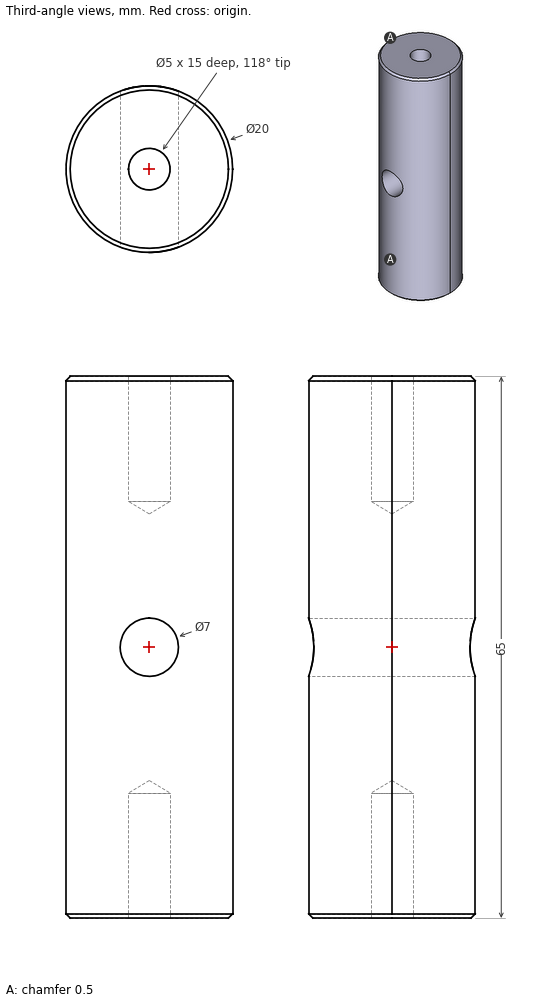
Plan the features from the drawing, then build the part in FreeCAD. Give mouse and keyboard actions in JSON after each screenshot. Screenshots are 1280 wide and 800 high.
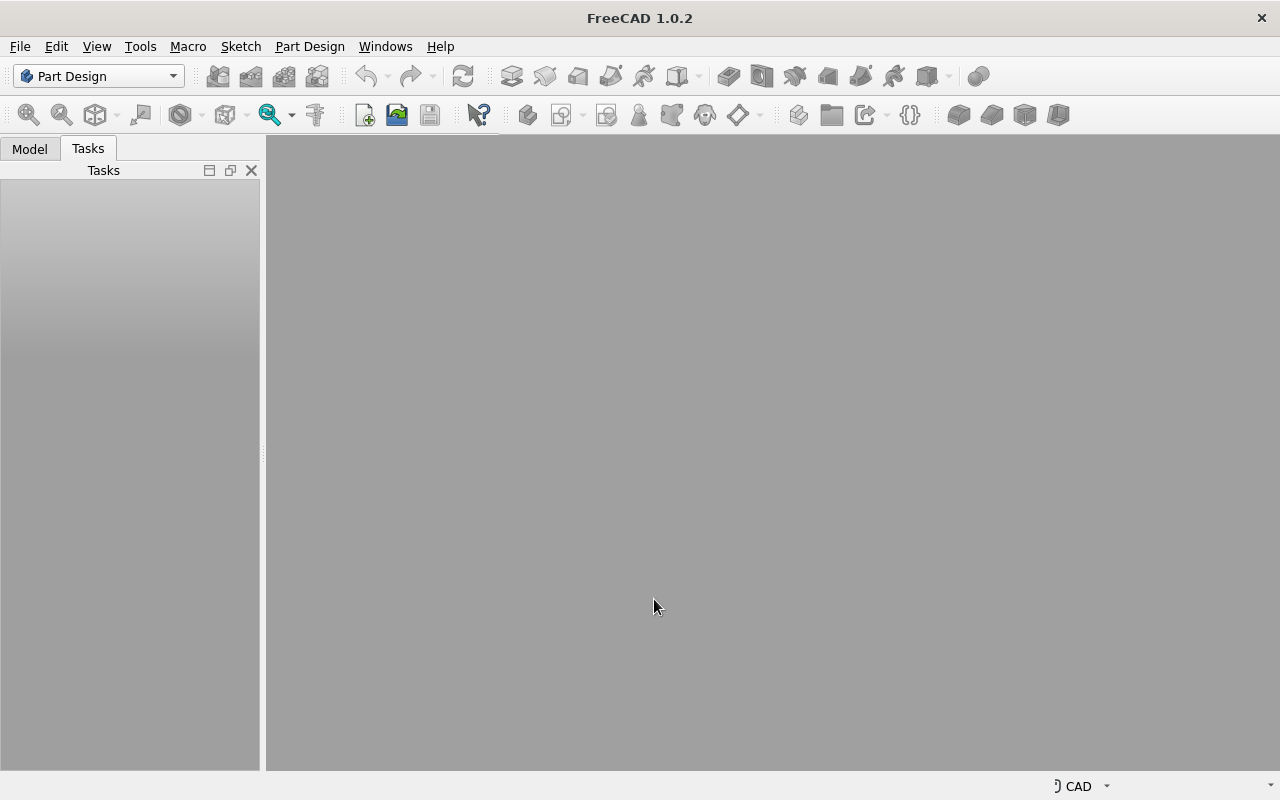
{"action": "left_click", "coordinate": [364, 116]}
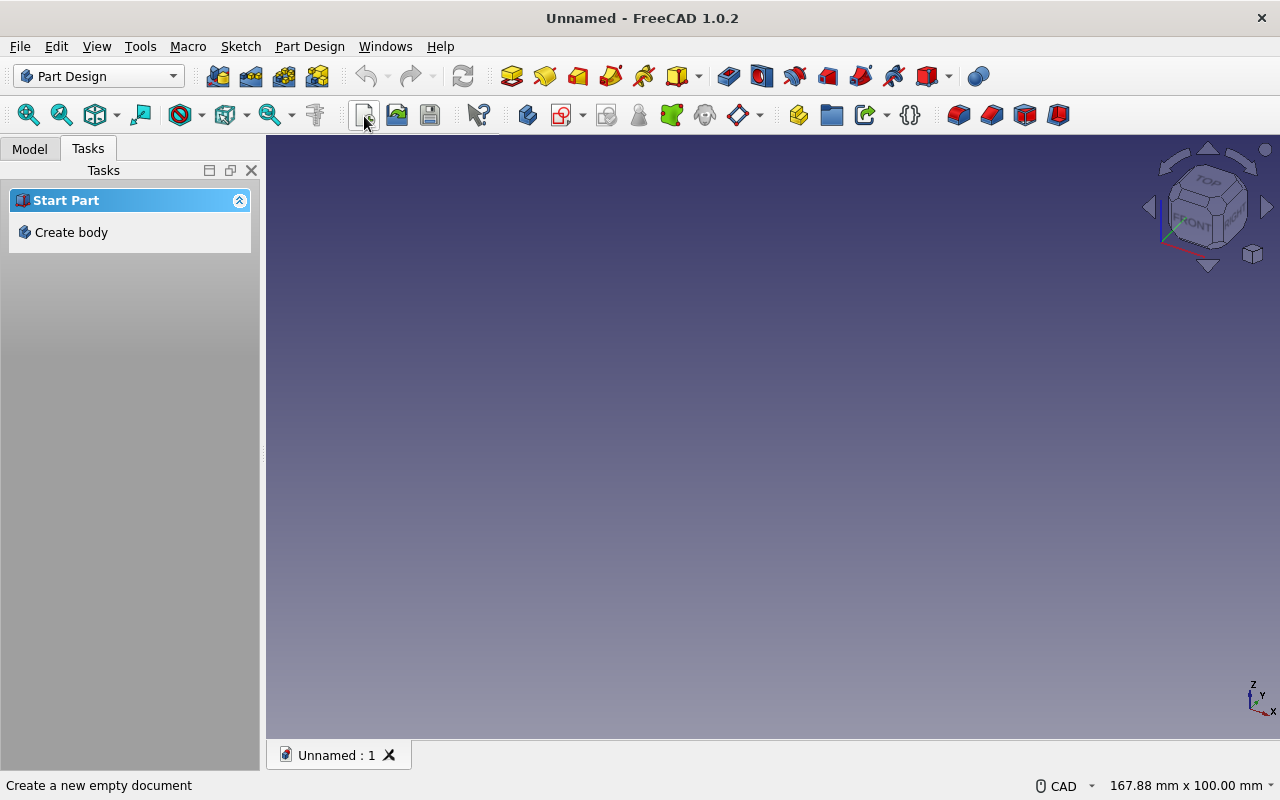
{"action": "left_click", "coordinate": [560, 116]}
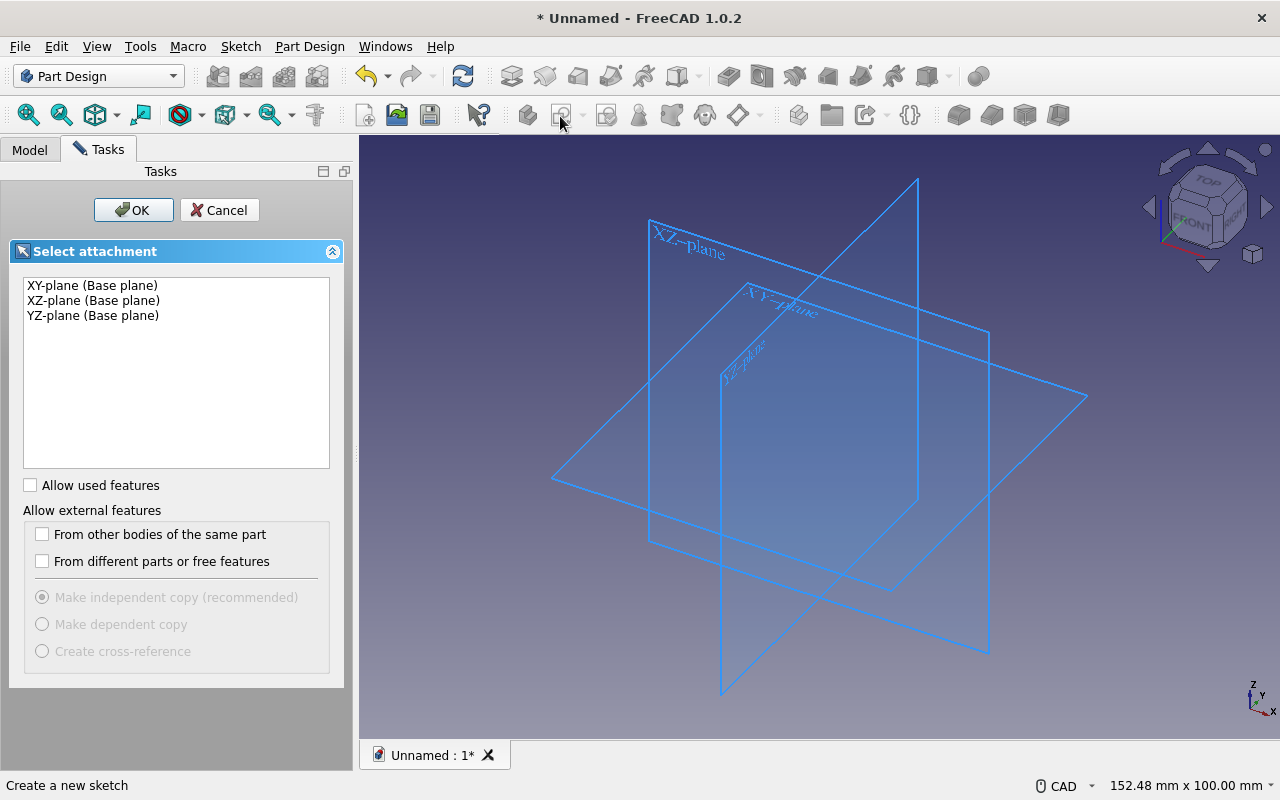
{"action": "left_click", "coordinate": [84, 286]}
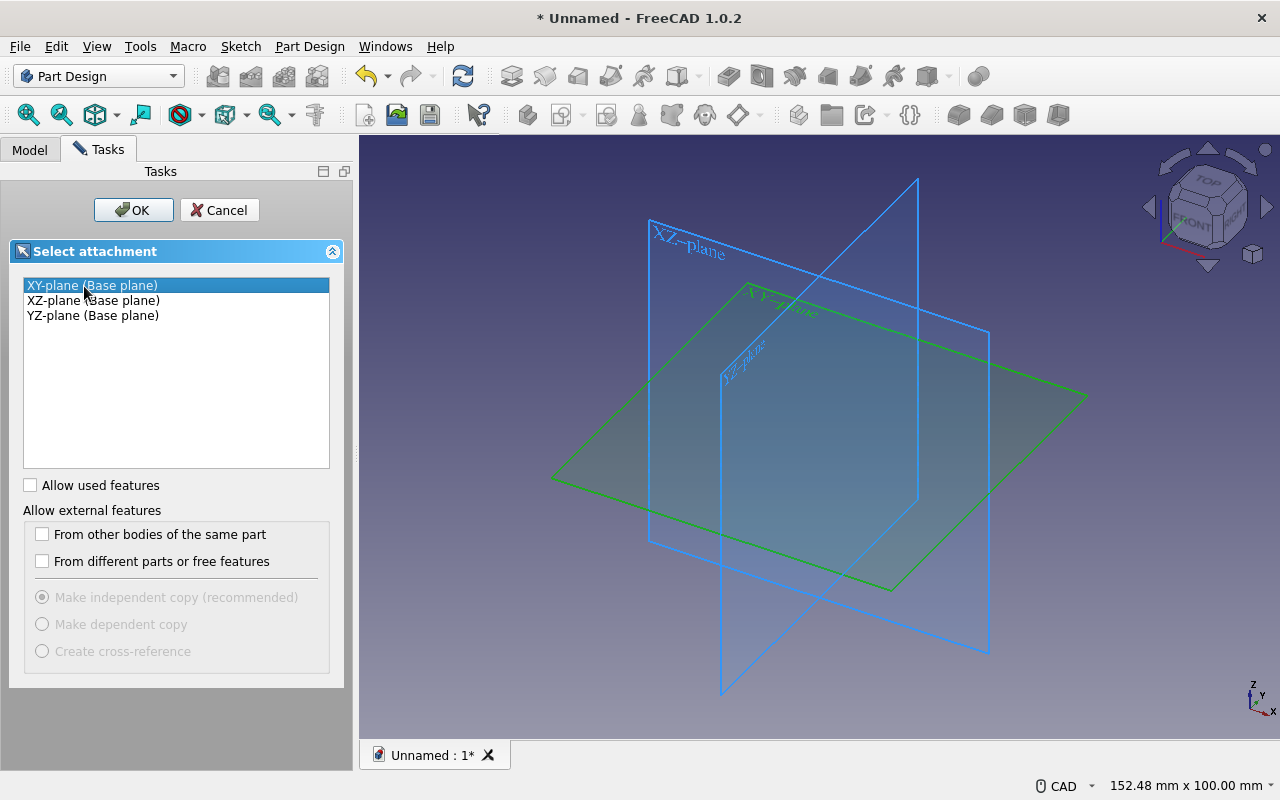
{"action": "left_click", "coordinate": [134, 210]}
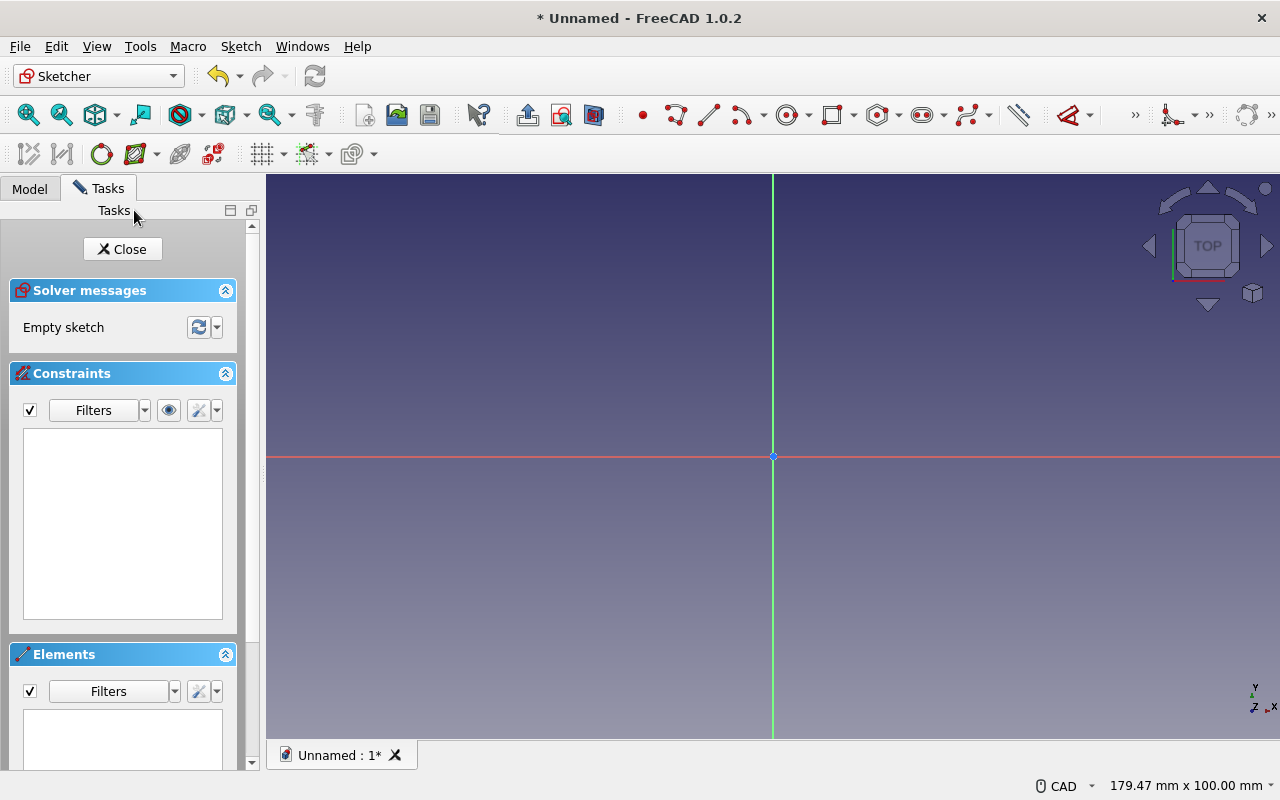
{"action": "scroll", "coordinate": [803, 456], "scroll_direction": "up", "scroll_amount": 6}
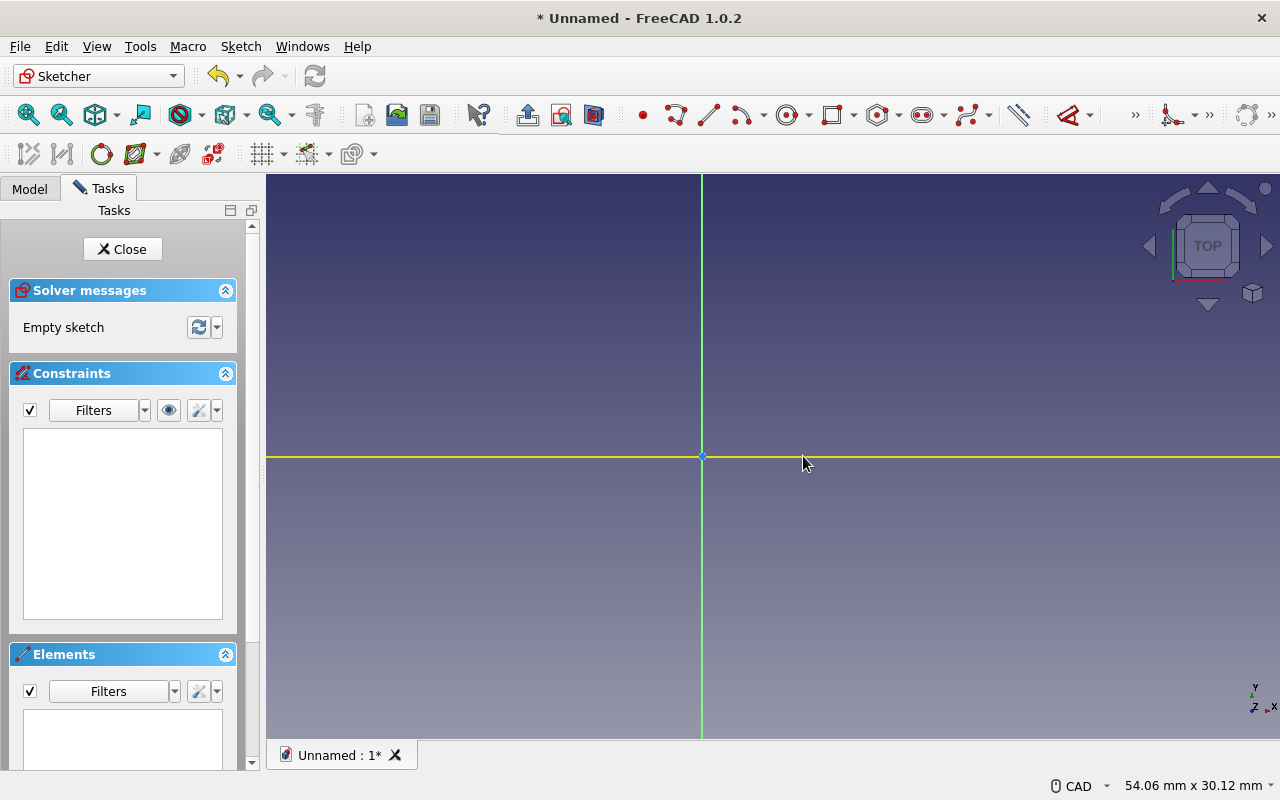
{"action": "left_click", "coordinate": [786, 116]}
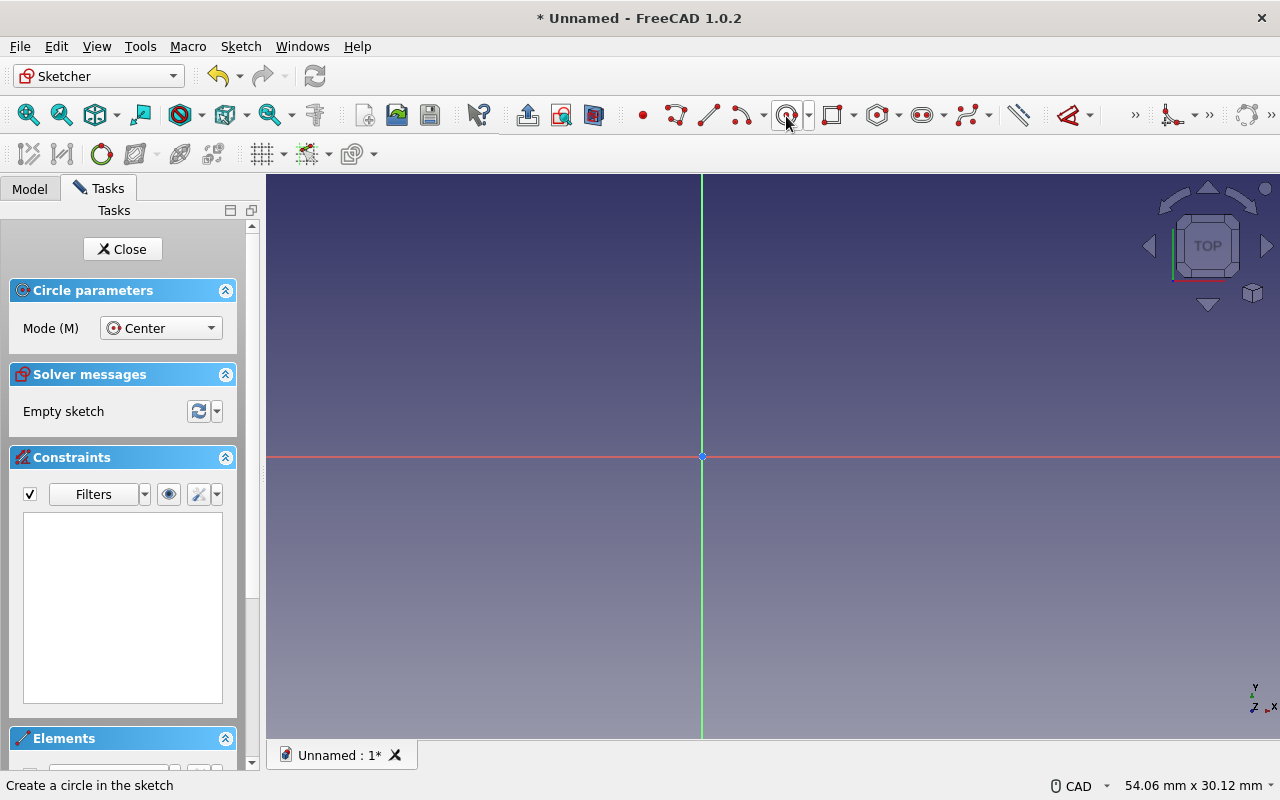
{"action": "left_click", "coordinate": [702, 456]}
{"action": "left_click", "coordinate": [835, 324]}
{"action": "key", "text": "Escape"}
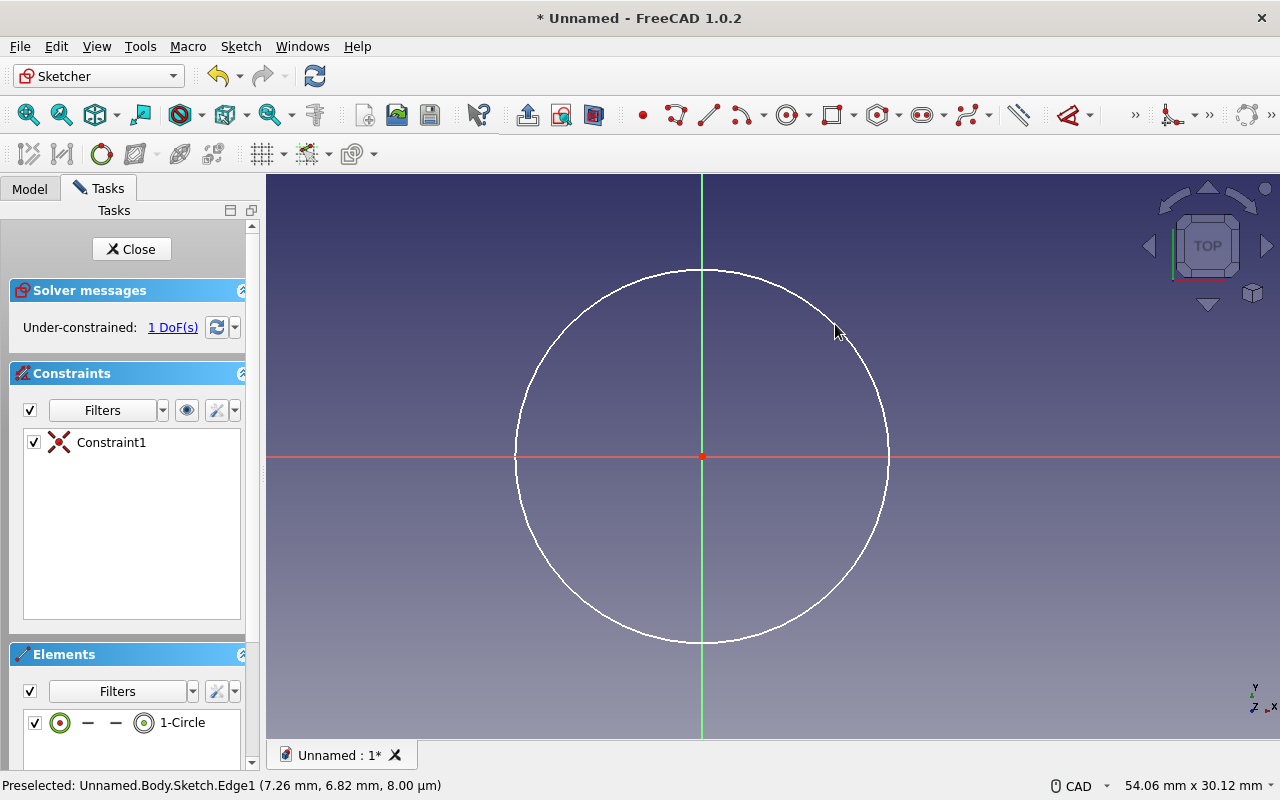
{"action": "left_click", "coordinate": [1068, 116]}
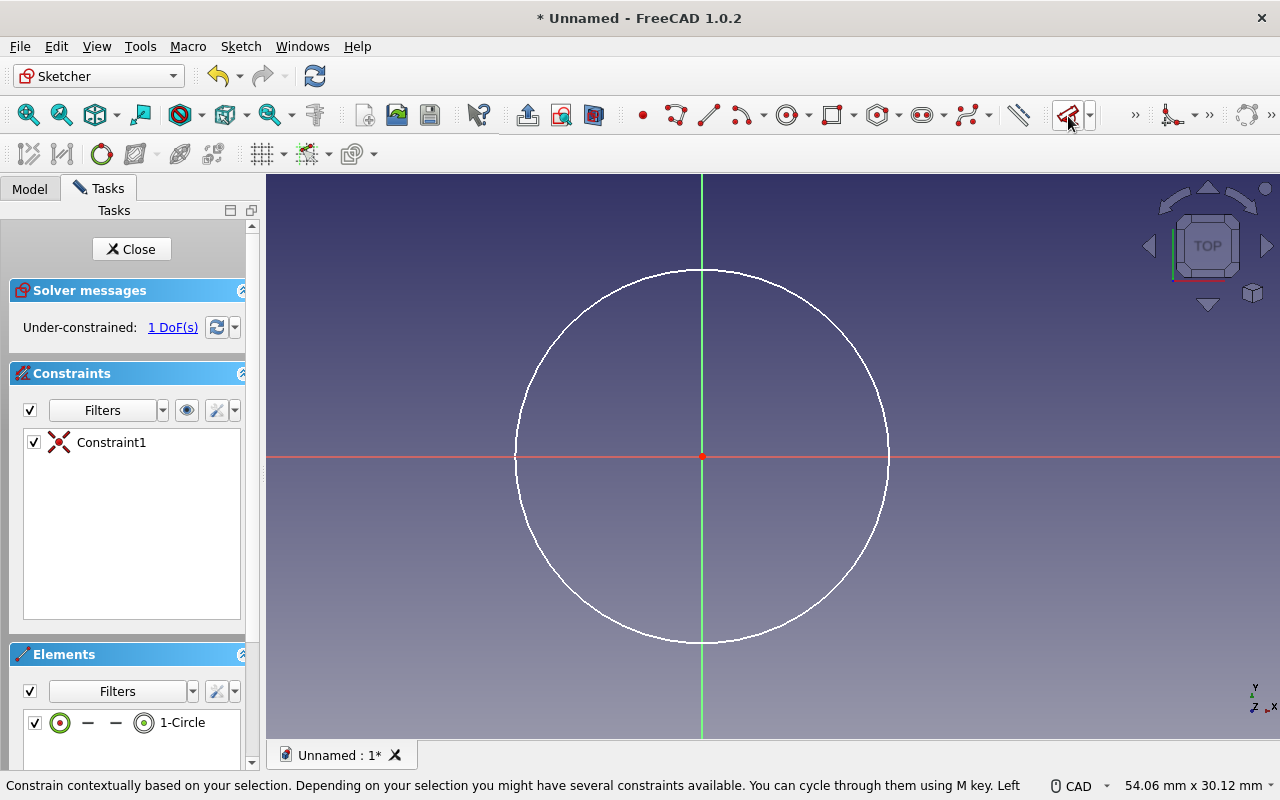
{"action": "left_click", "coordinate": [834, 324]}
{"action": "left_click", "coordinate": [857, 301]}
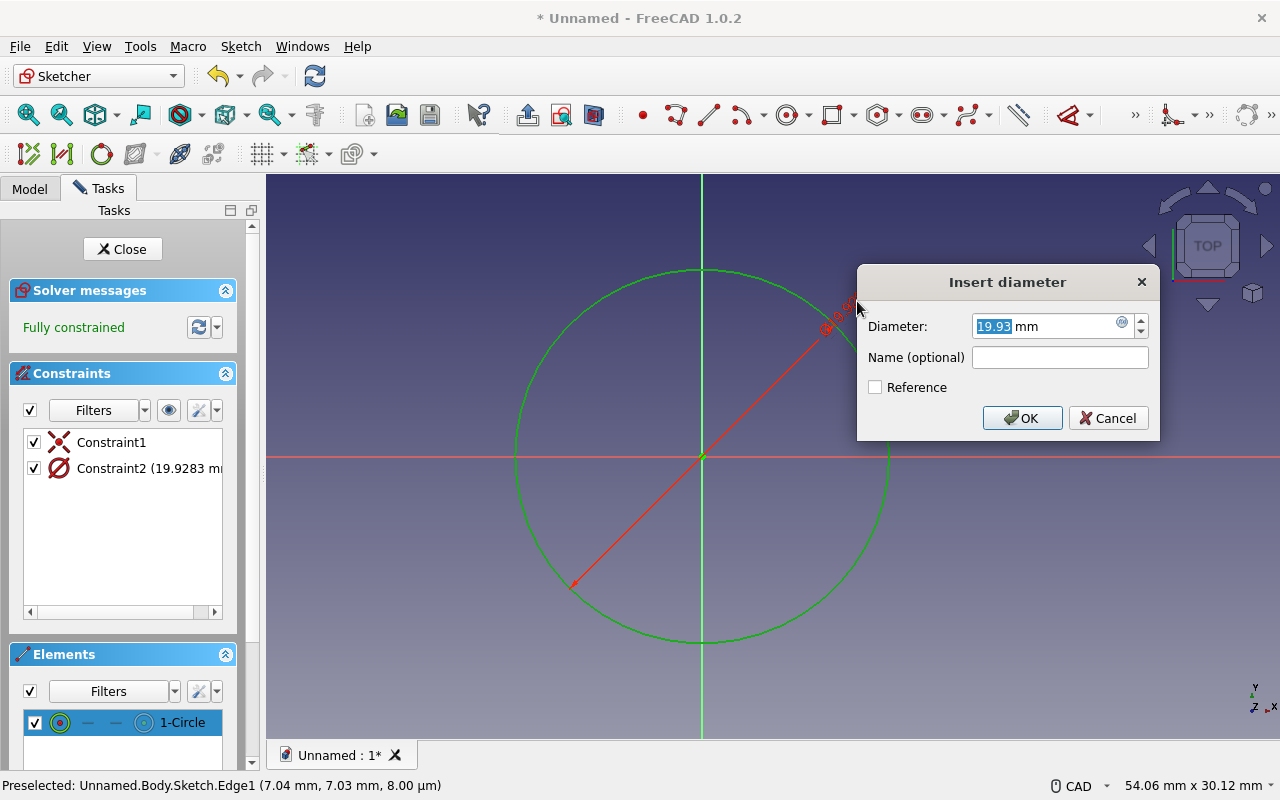
{"action": "type", "text": "20"}
{"action": "key", "text": "Return"}
{"action": "key", "text": "Escape"}